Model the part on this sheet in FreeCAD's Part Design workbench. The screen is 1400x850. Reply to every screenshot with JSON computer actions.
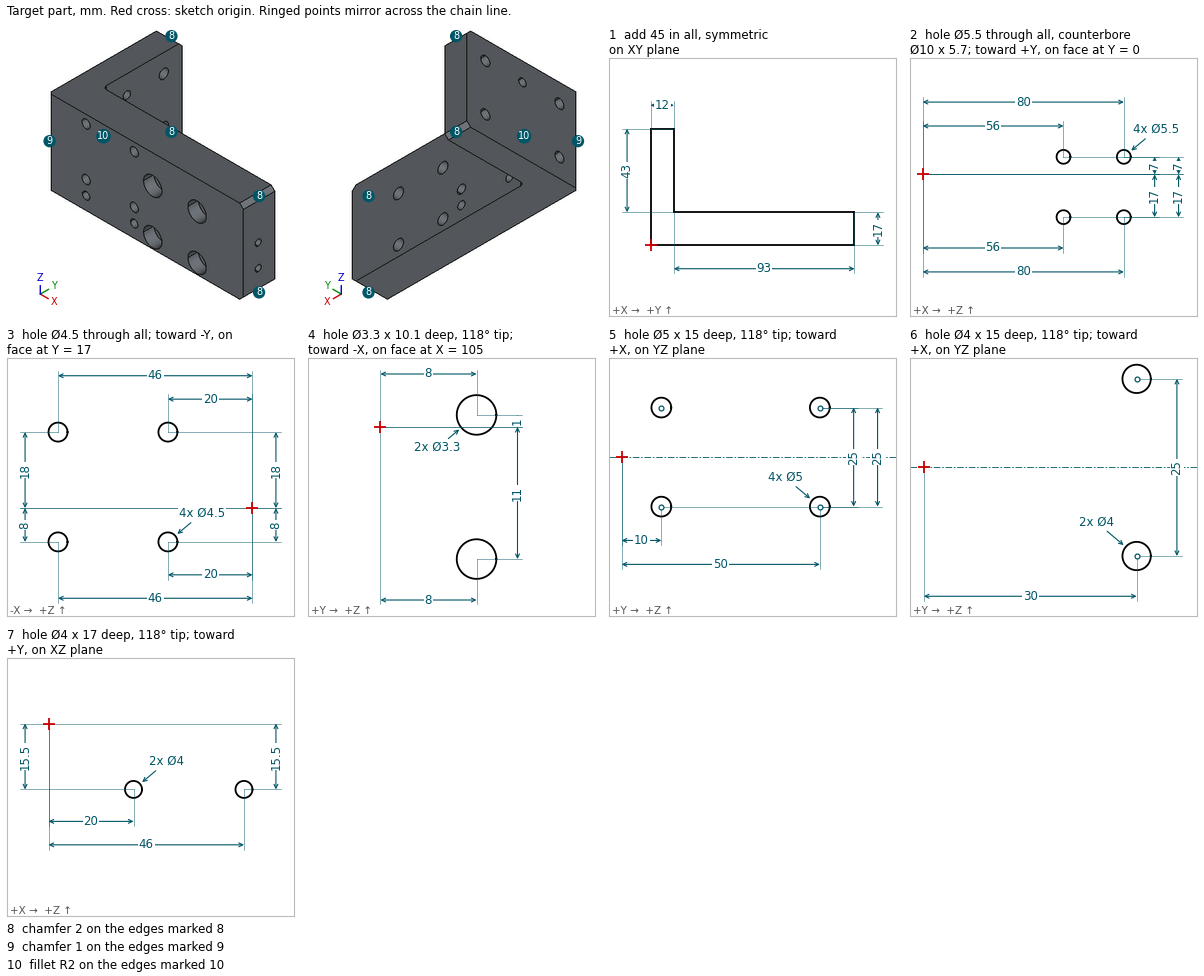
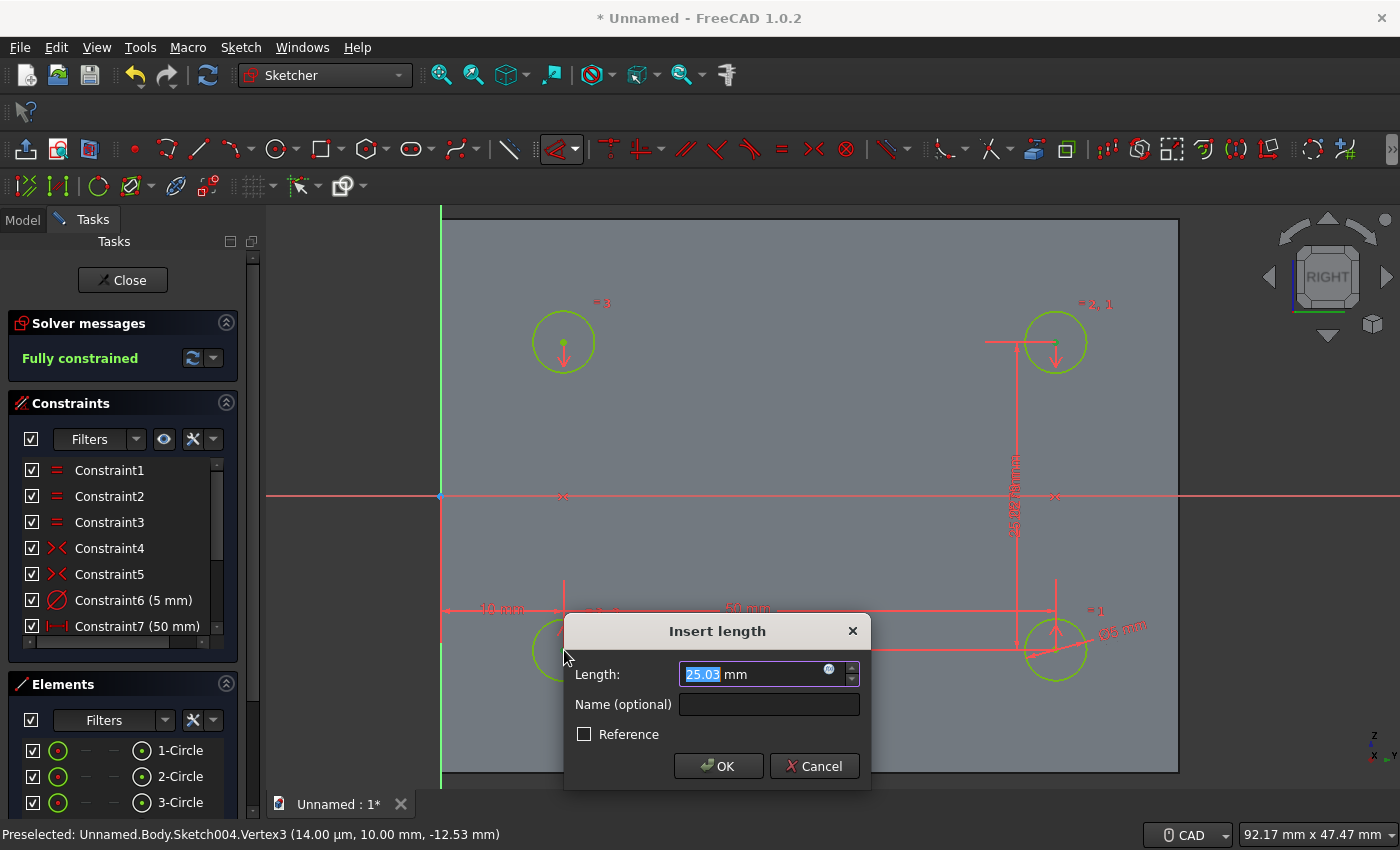
{"action": "type", "text": "25"}
{"action": "key", "text": "Return"}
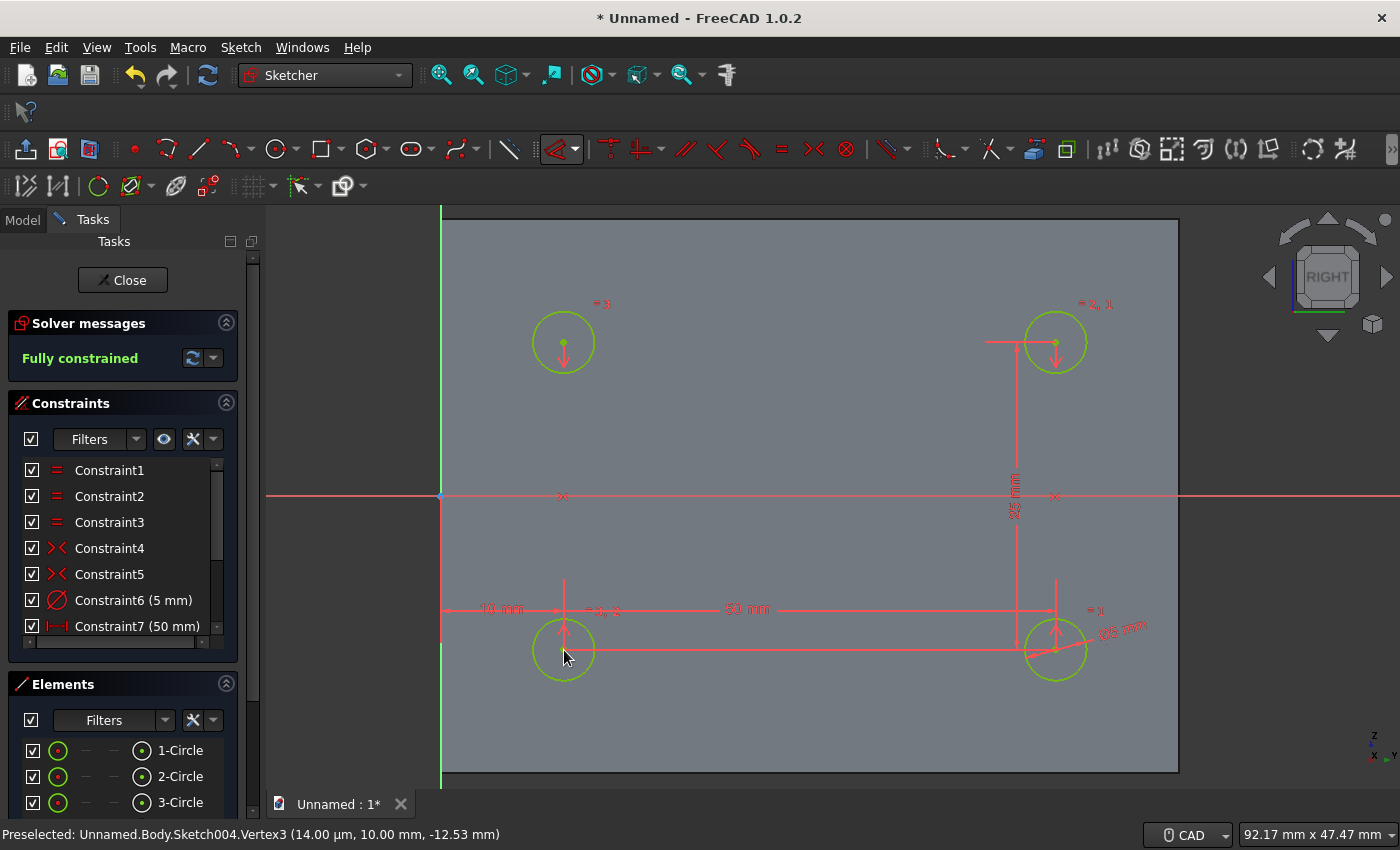
{"action": "left_click", "coordinate": [123, 280]}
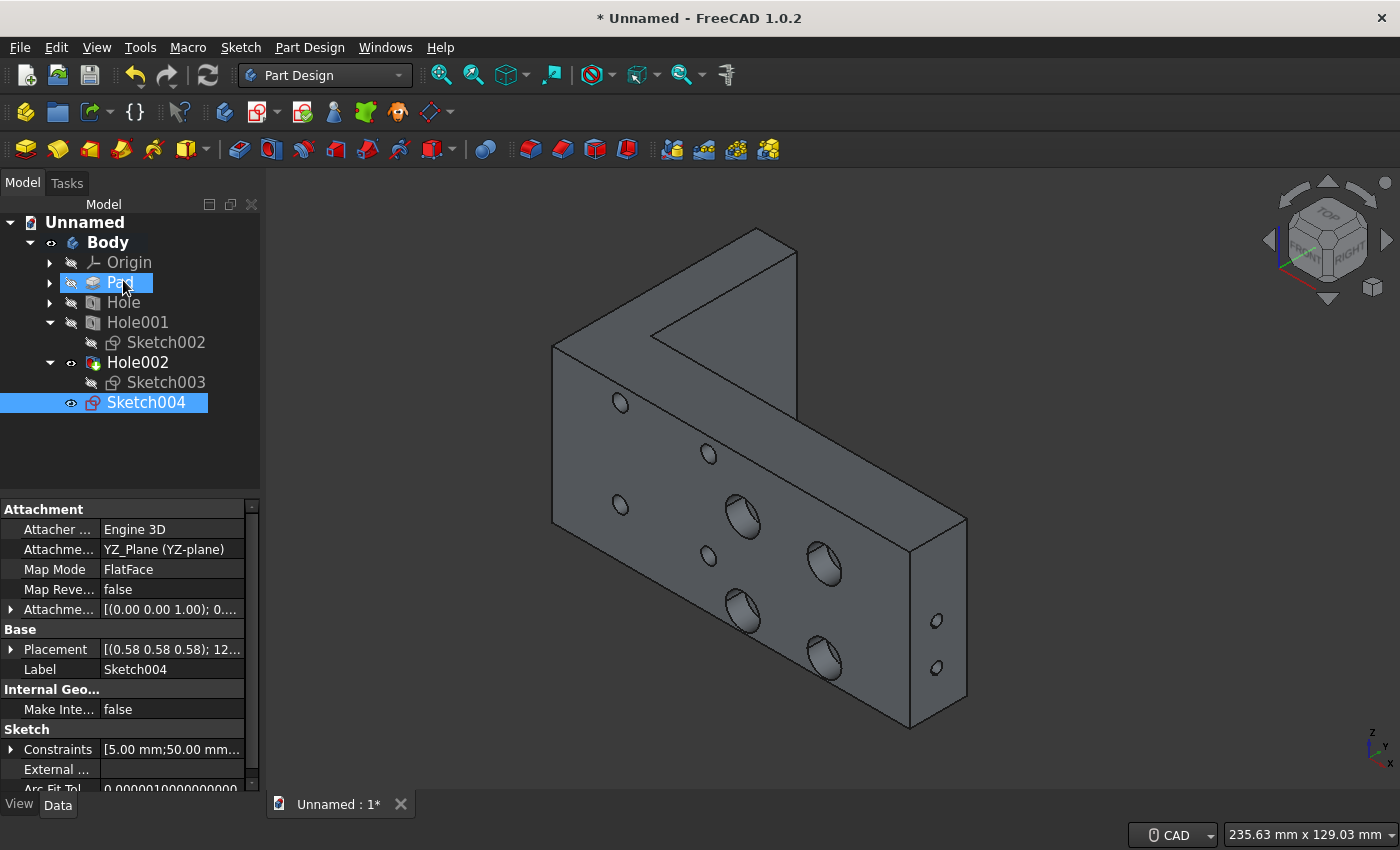
{"action": "left_click", "coordinate": [272, 150]}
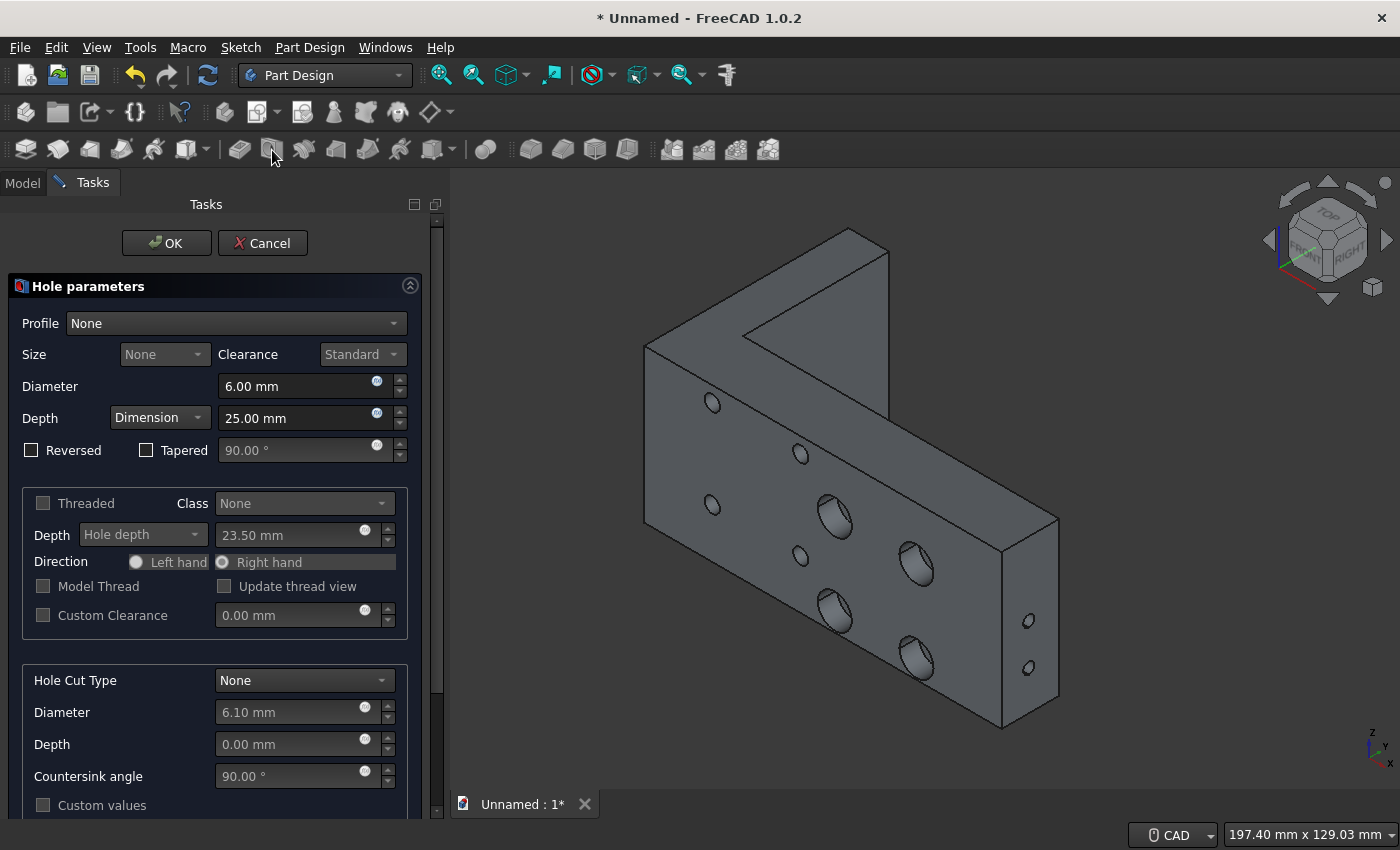
{"action": "triple_click", "coordinate": [305, 386]}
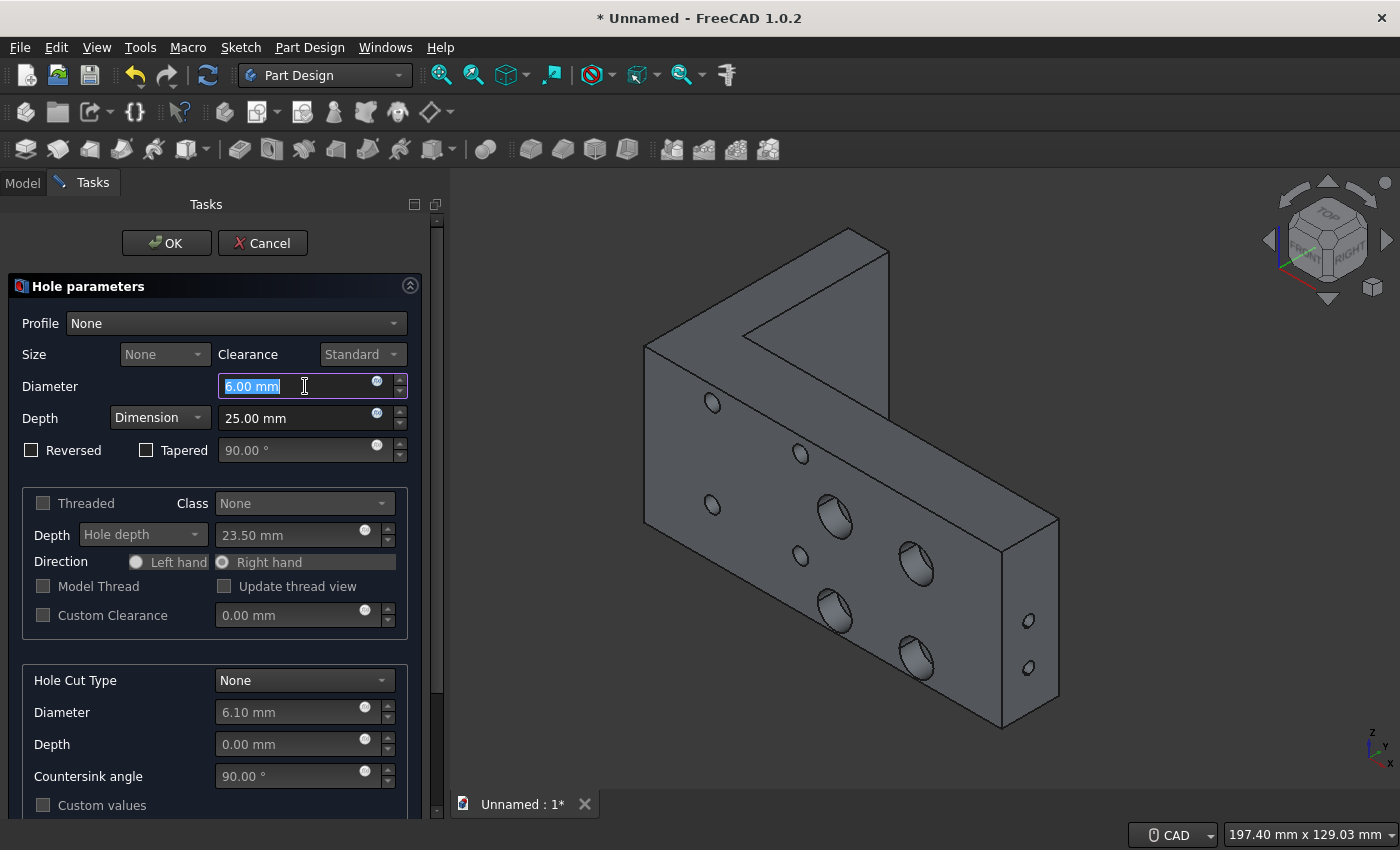
{"action": "type", "text": "5"}
{"action": "key", "text": "Tab"}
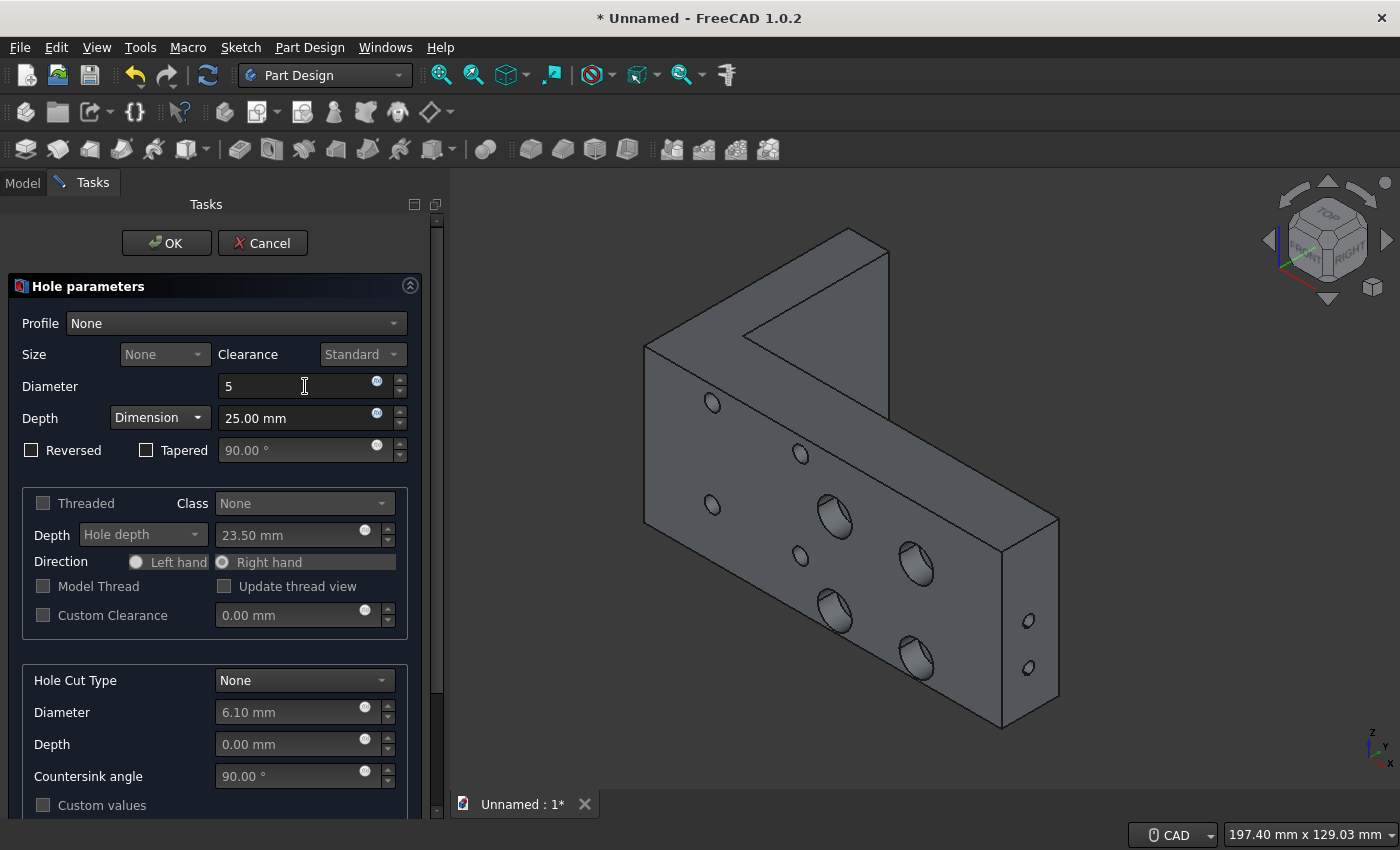
{"action": "triple_click", "coordinate": [305, 418]}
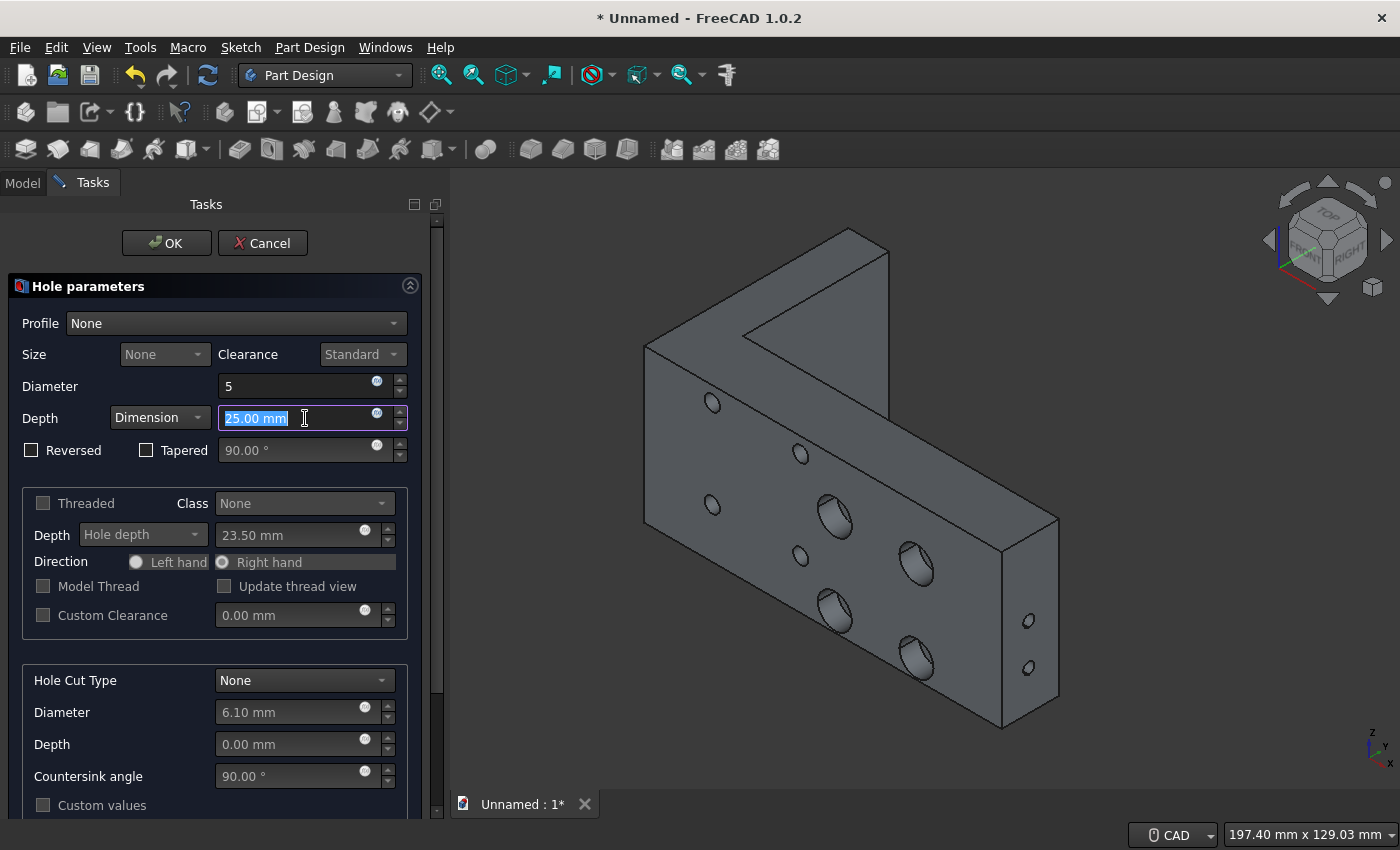
{"action": "type", "text": "15"}
{"action": "key", "text": "Tab"}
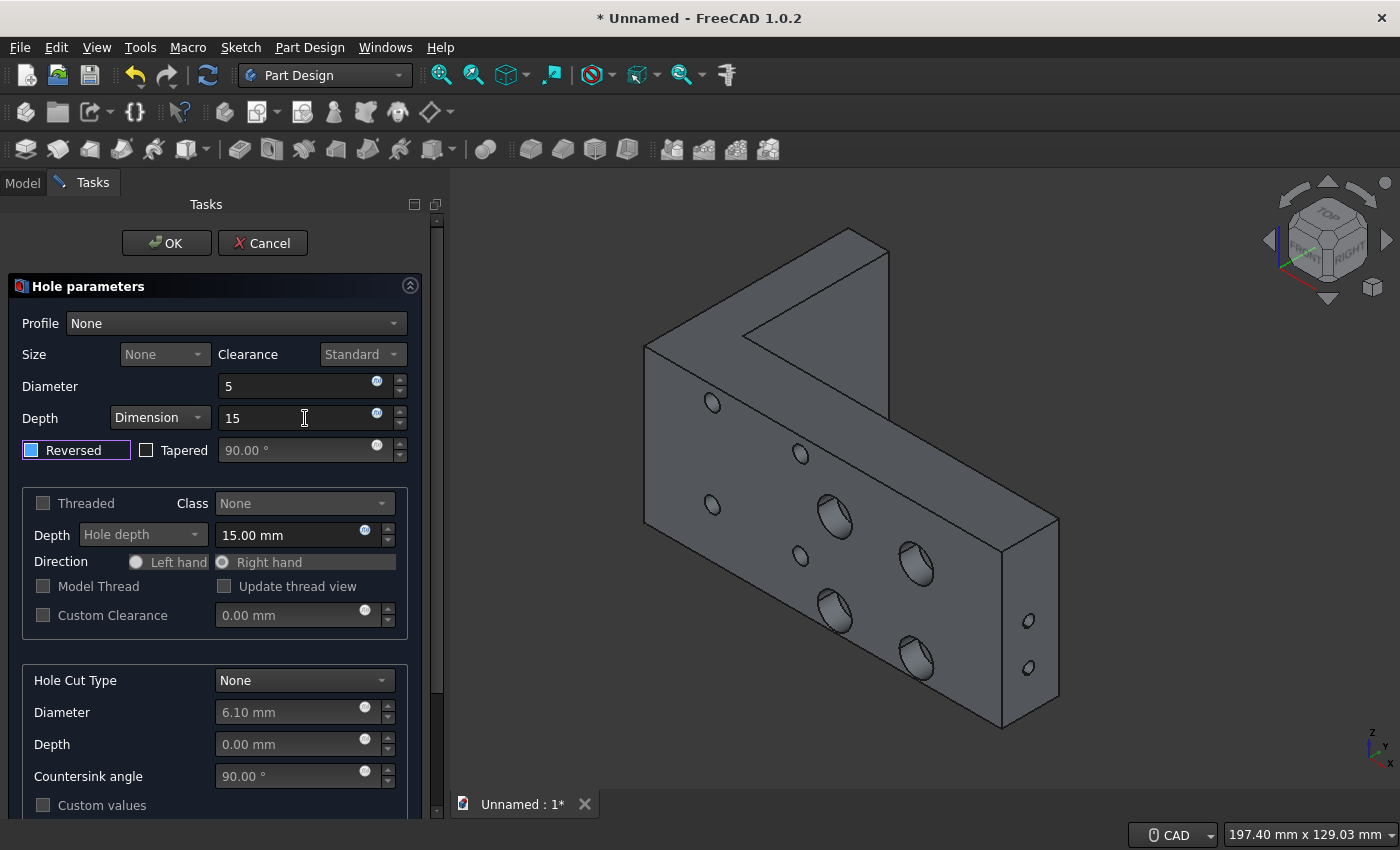
{"action": "left_click", "coordinate": [30, 450]}